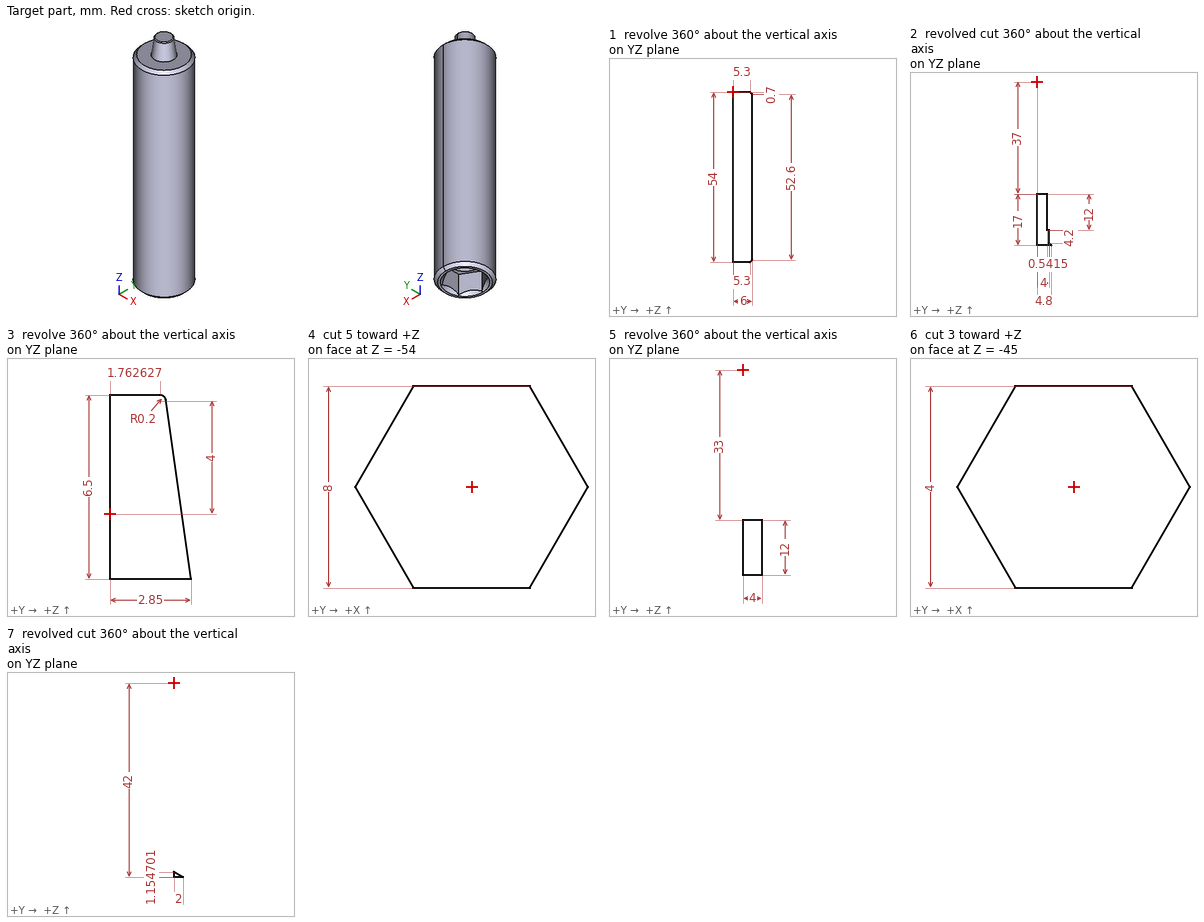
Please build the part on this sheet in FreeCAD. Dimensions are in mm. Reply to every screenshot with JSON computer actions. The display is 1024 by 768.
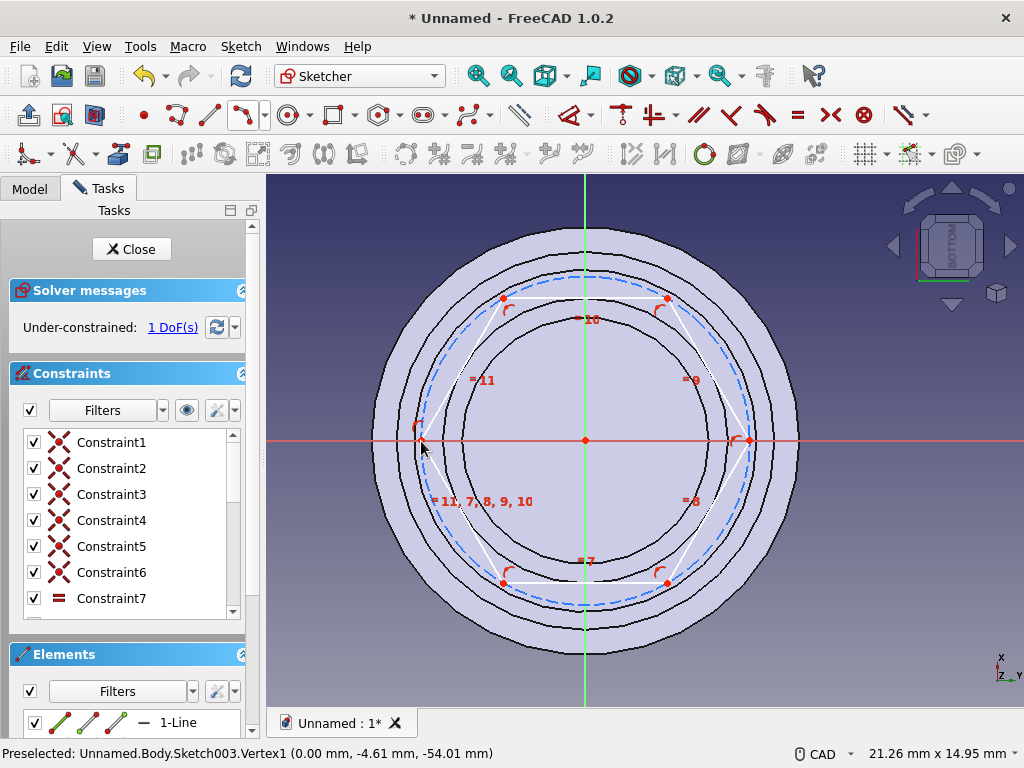
{"action": "left_click", "coordinate": [568, 116]}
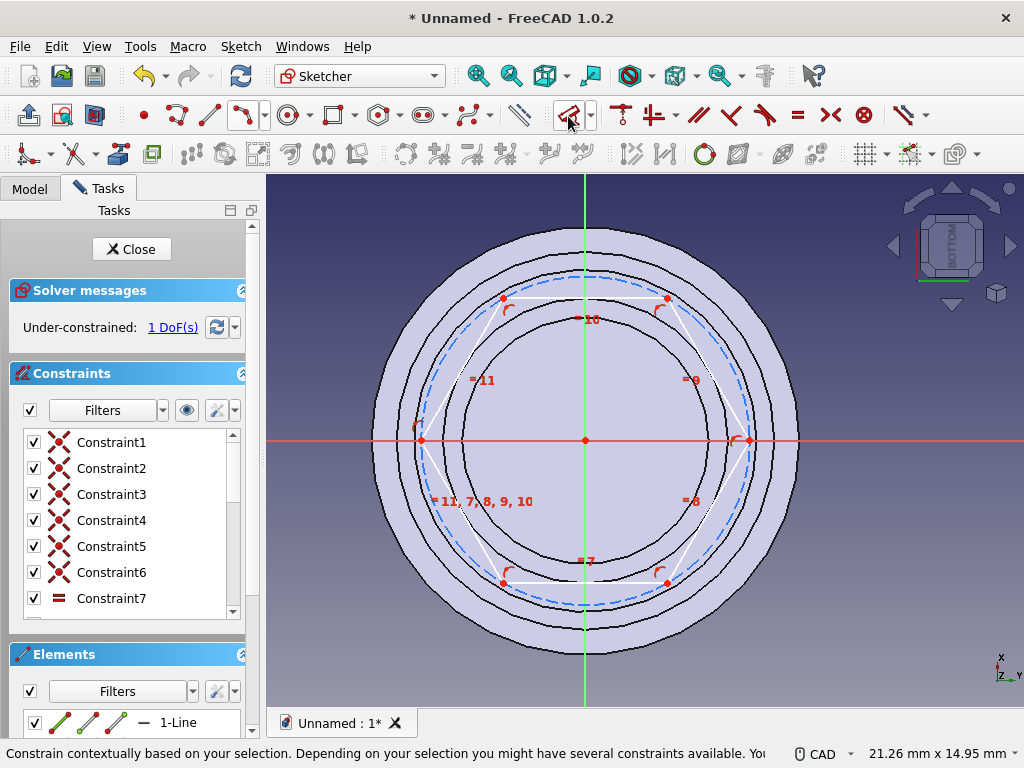
{"action": "left_click", "coordinate": [503, 583]}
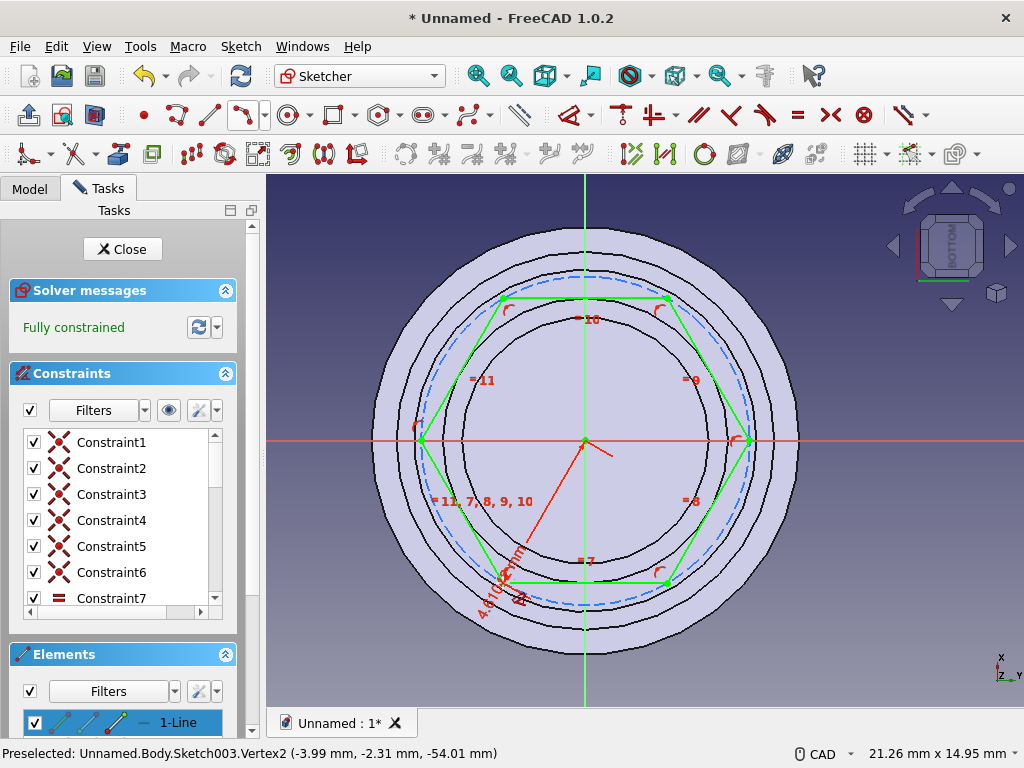
{"action": "left_click", "coordinate": [668, 298]}
{"action": "left_click", "coordinate": [750, 341]}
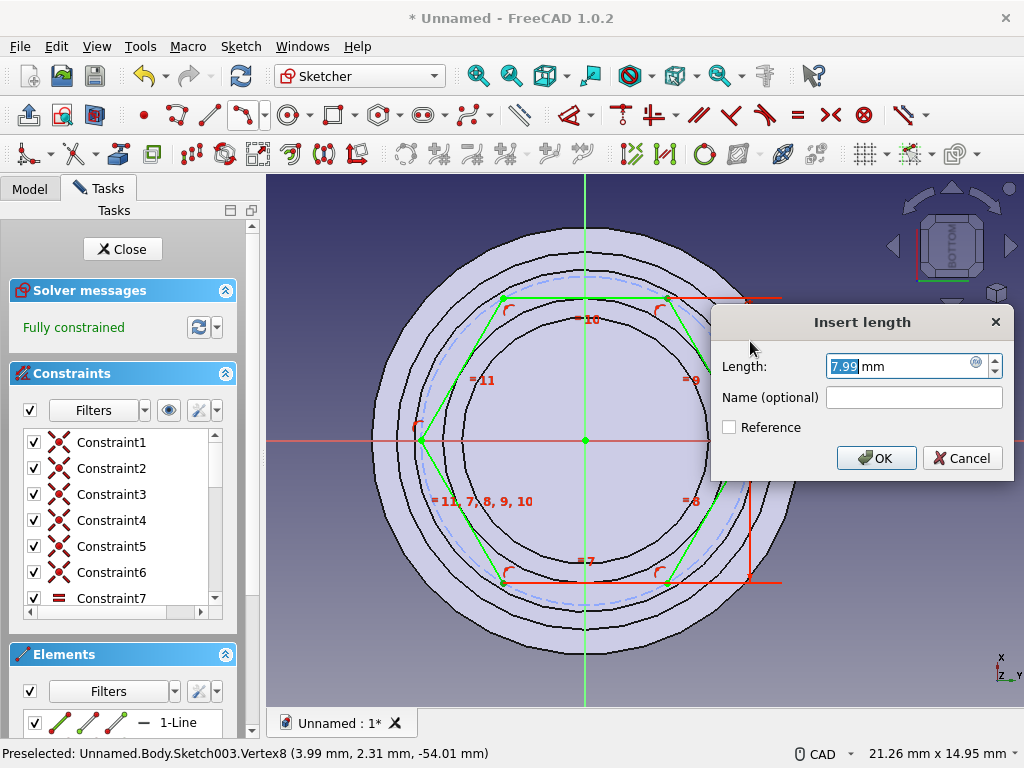
{"action": "type", "text": "8"}
{"action": "key", "text": "Return"}
{"action": "key", "text": "Escape"}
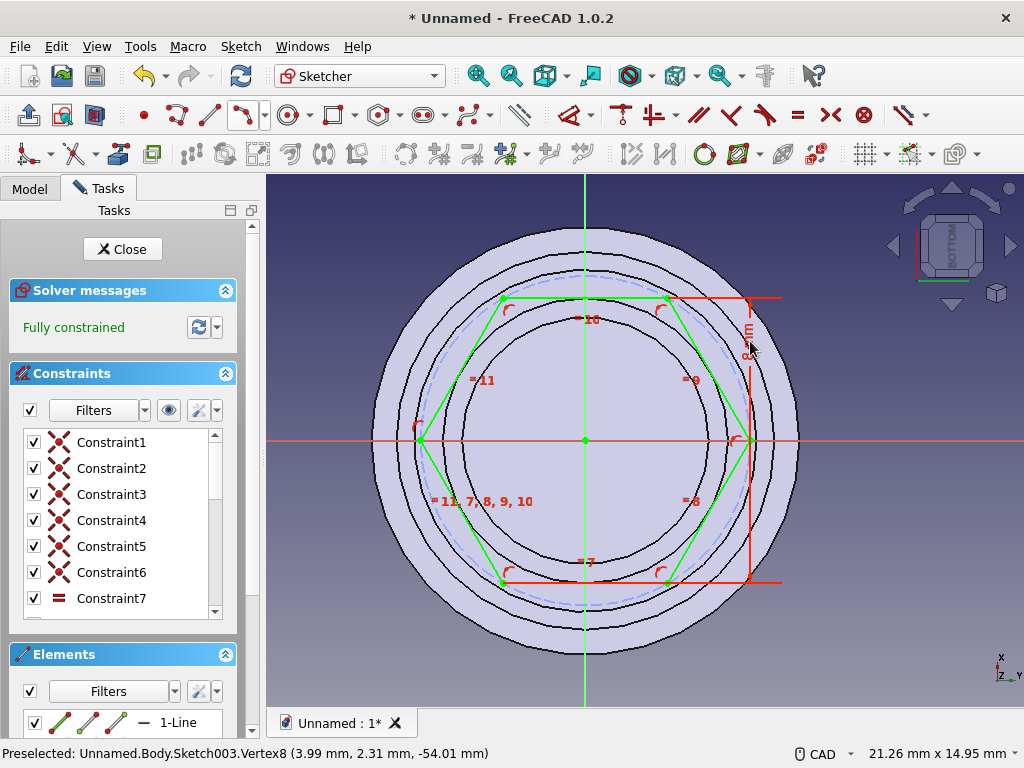
{"action": "left_click", "coordinate": [123, 249]}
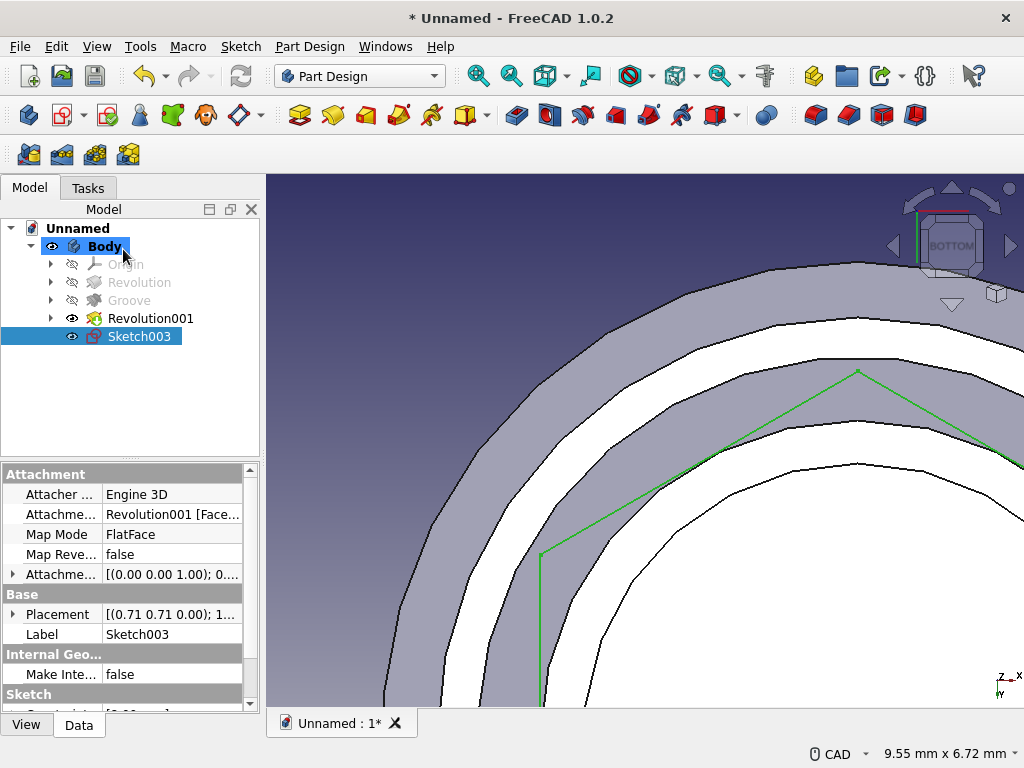
{"action": "left_click", "coordinate": [517, 116]}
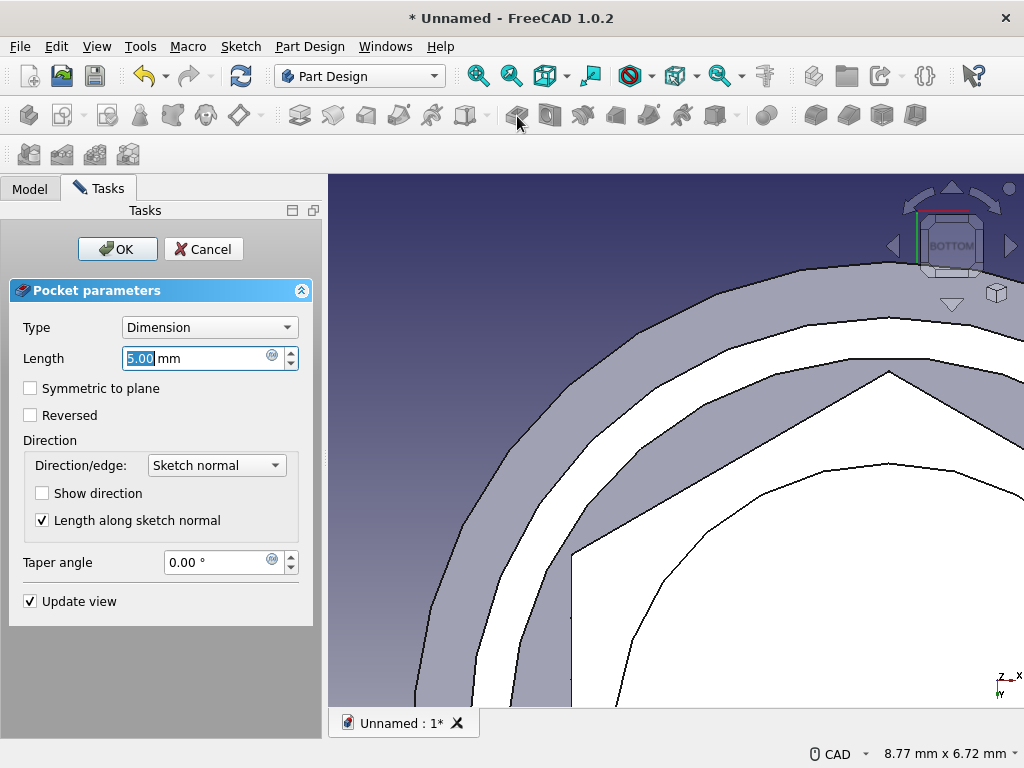
{"action": "type", "text": "5"}
{"action": "key", "text": "Tab"}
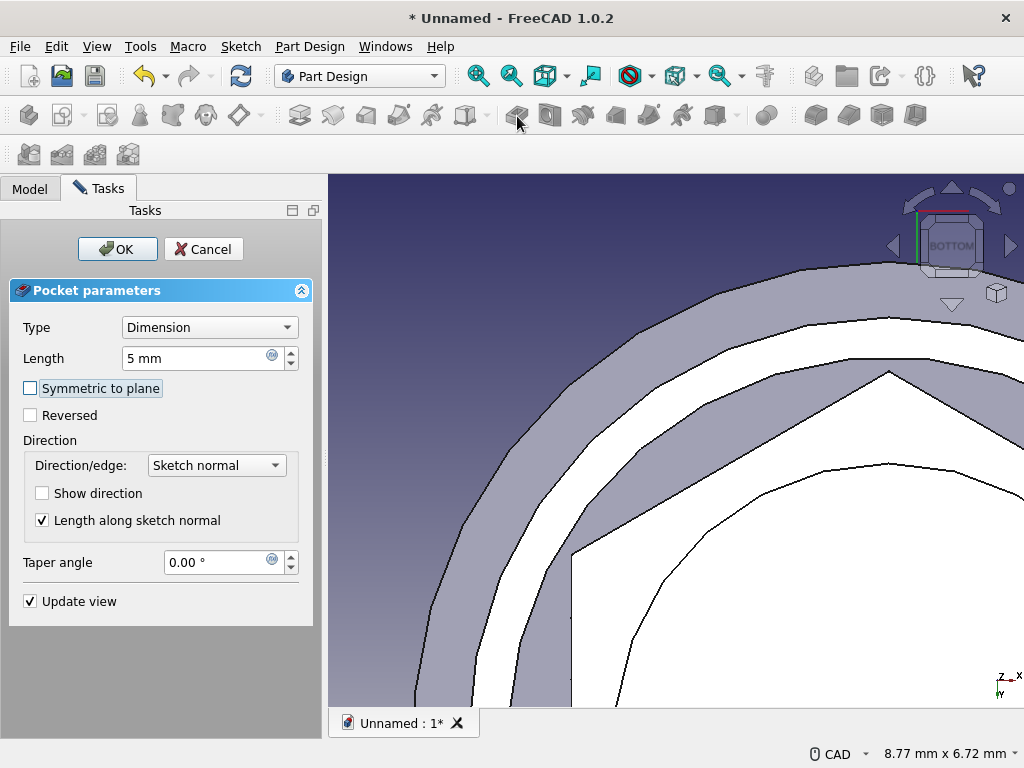
{"action": "left_click", "coordinate": [118, 249]}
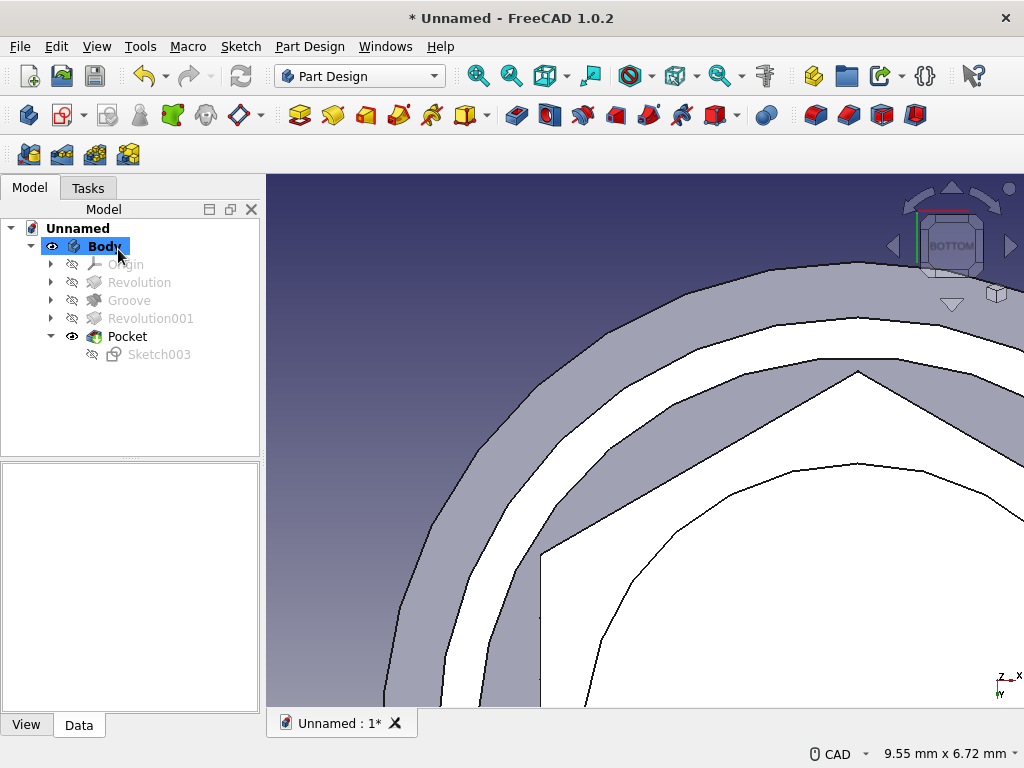
{"action": "left_click", "coordinate": [479, 76]}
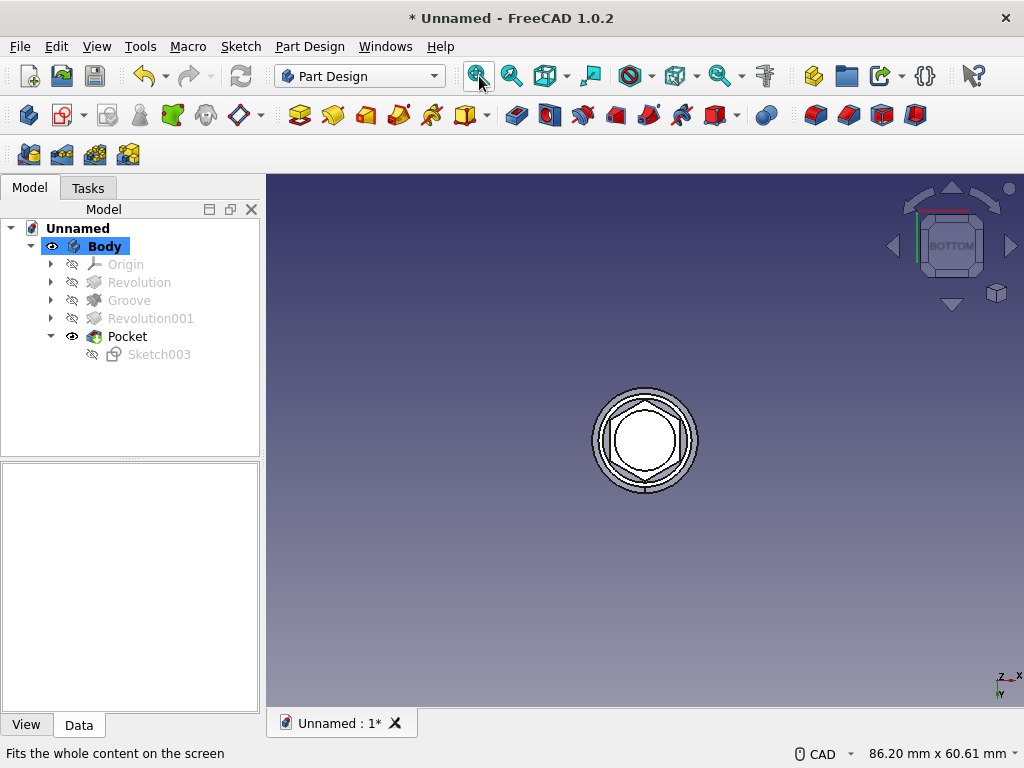
{"action": "left_click", "coordinate": [62, 116]}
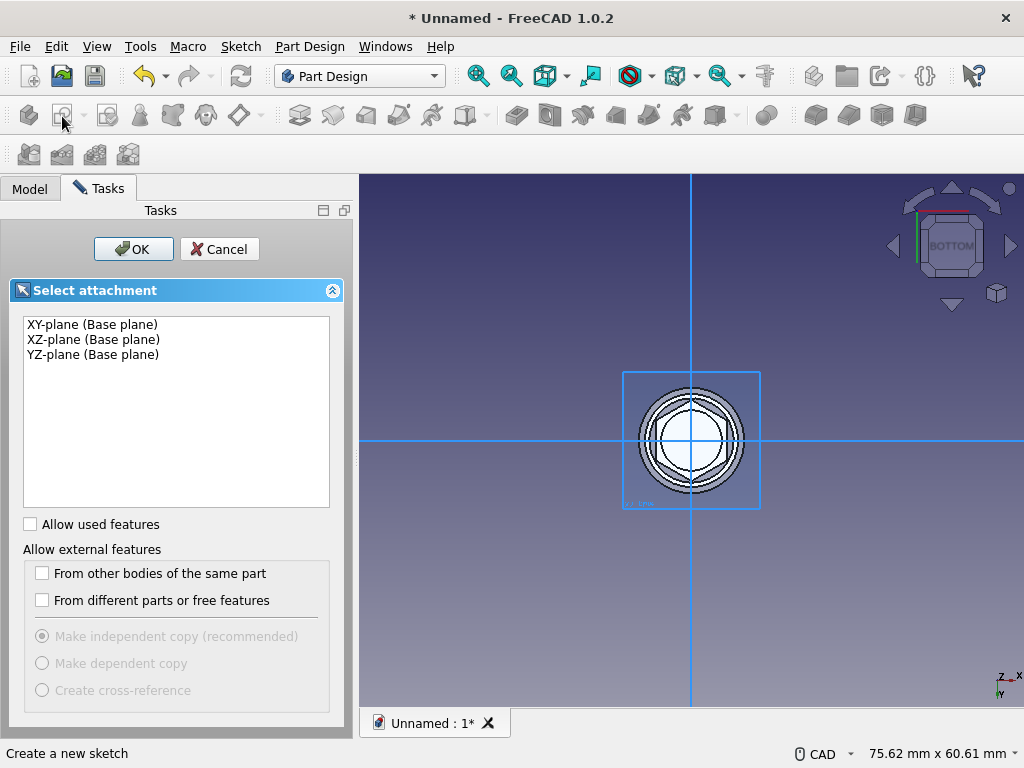
{"action": "left_click", "coordinate": [84, 354]}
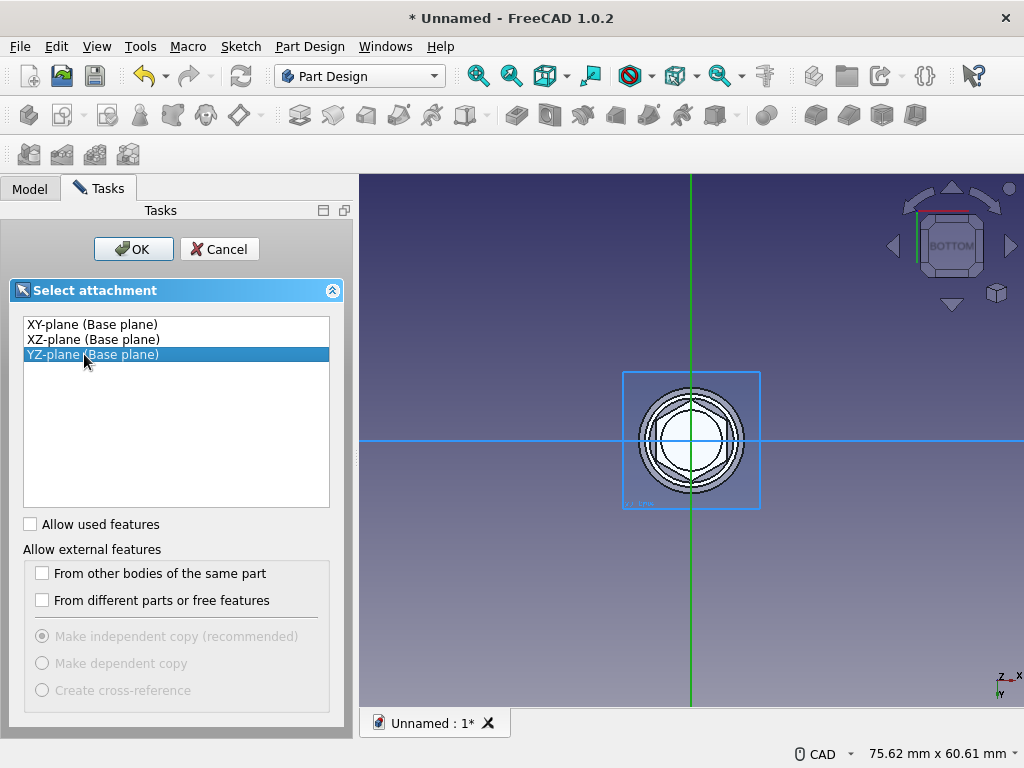
{"action": "left_click", "coordinate": [134, 249]}